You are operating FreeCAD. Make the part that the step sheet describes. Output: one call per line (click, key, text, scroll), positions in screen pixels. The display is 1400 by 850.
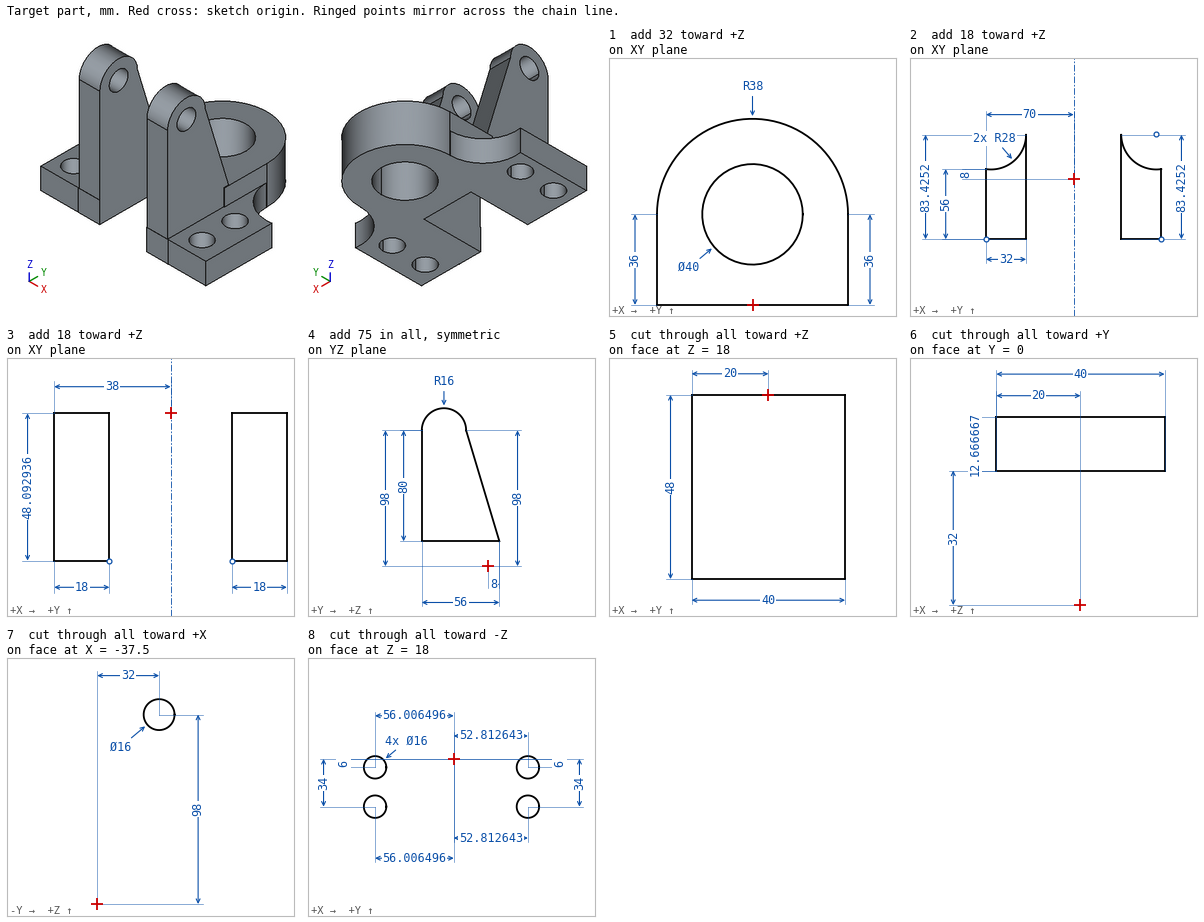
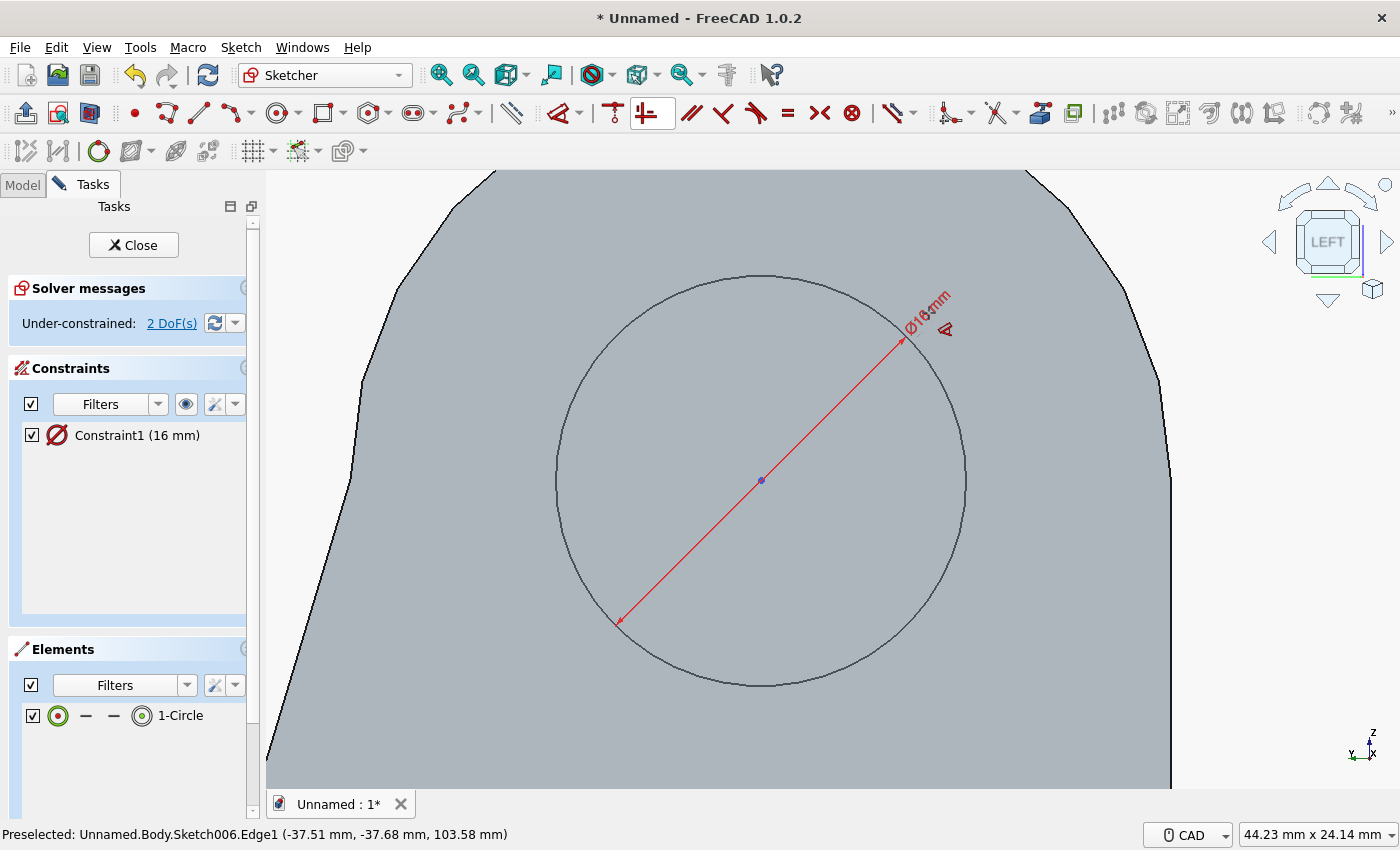
click(761, 481)
click(527, 447)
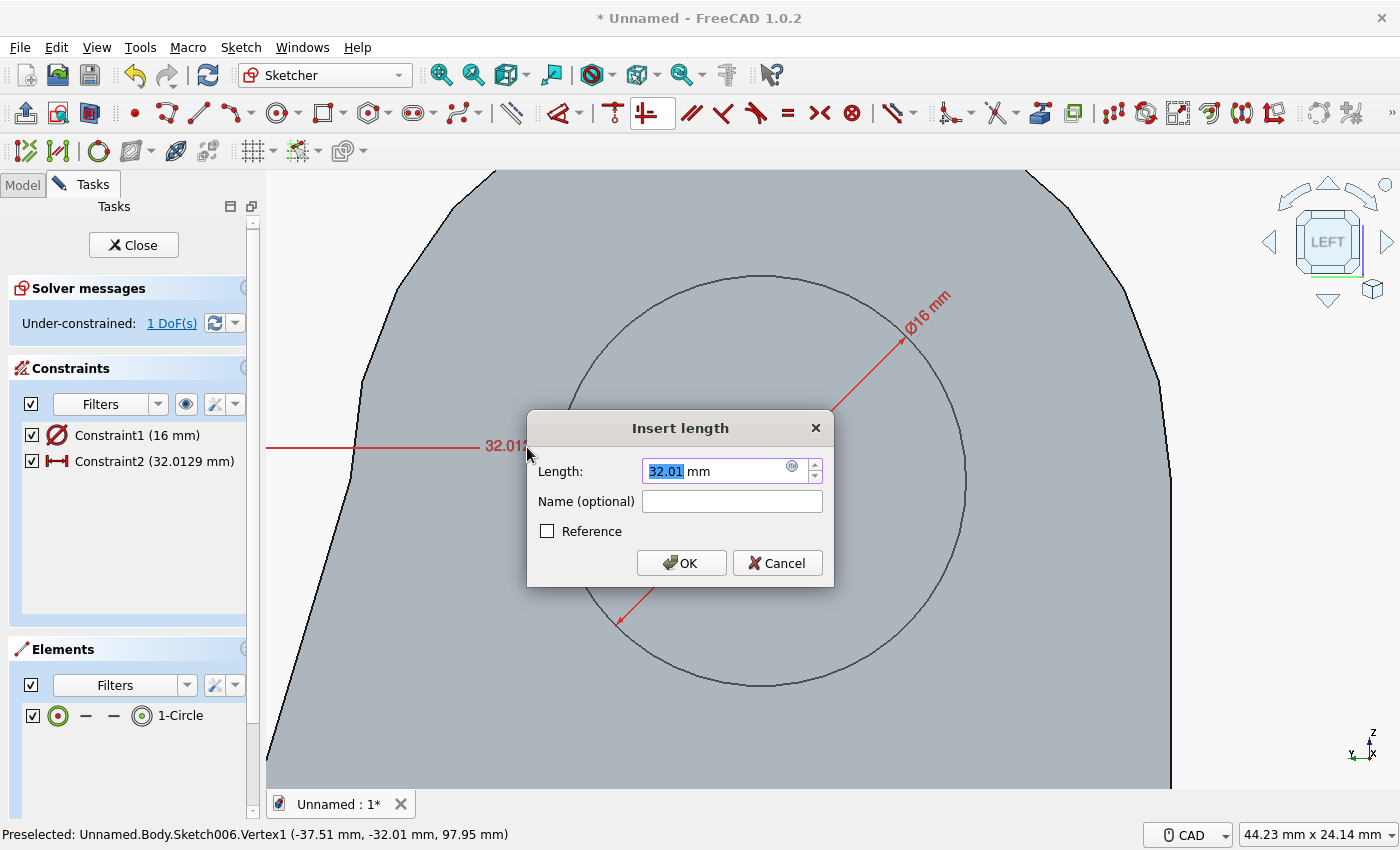
text(32)
key(Return)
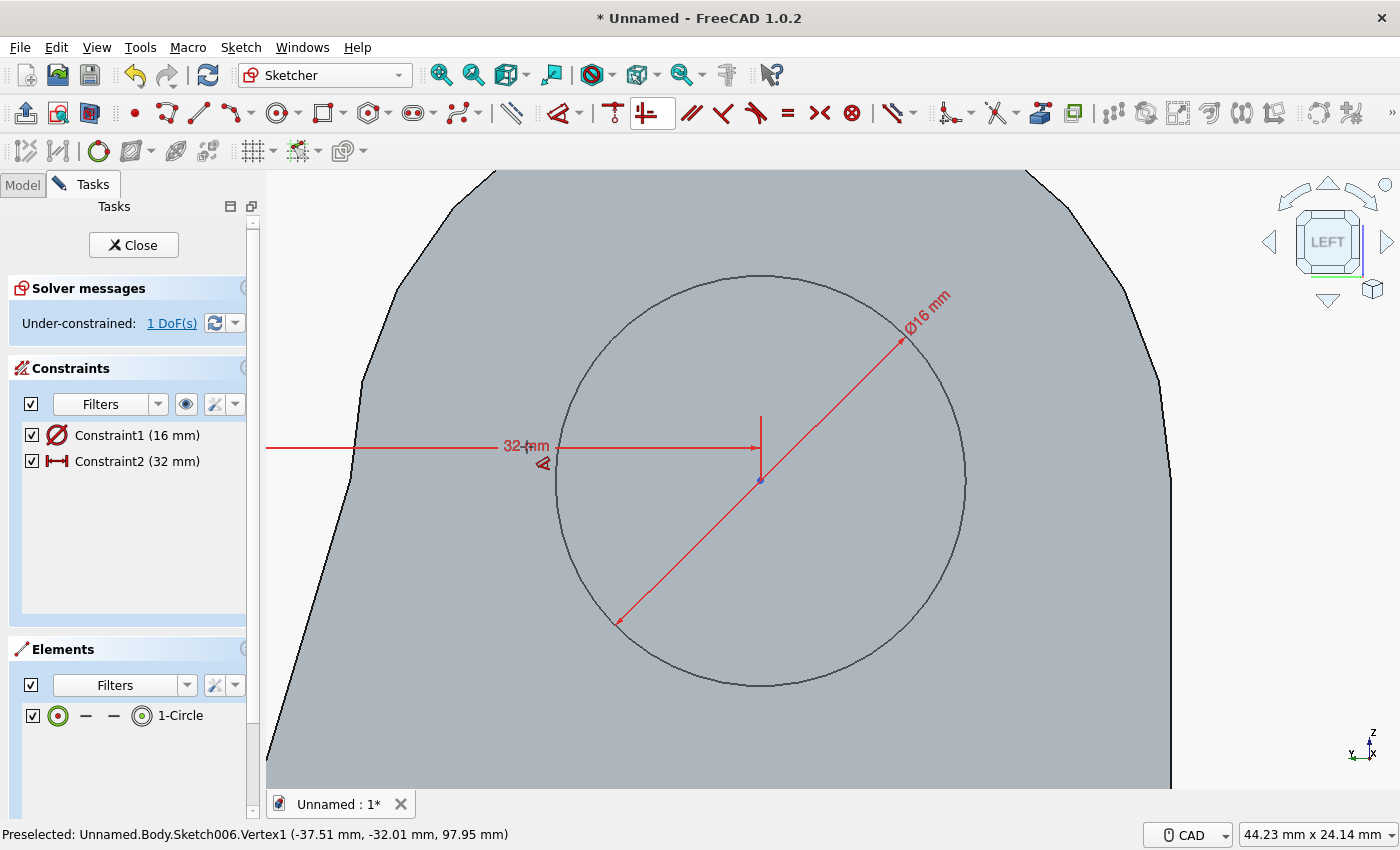
click(761, 481)
click(795, 621)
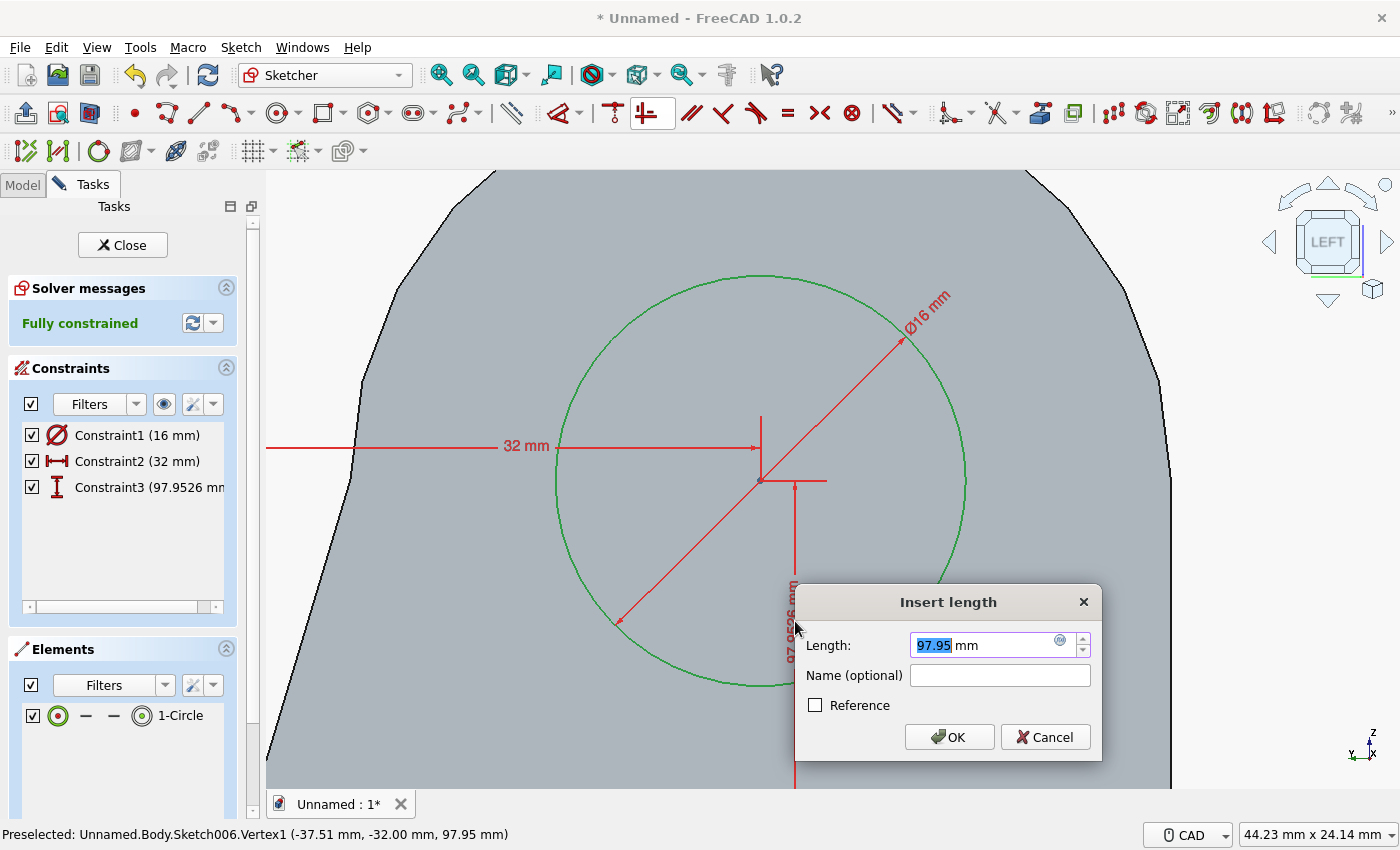
text(98)
key(Return)
key(Escape)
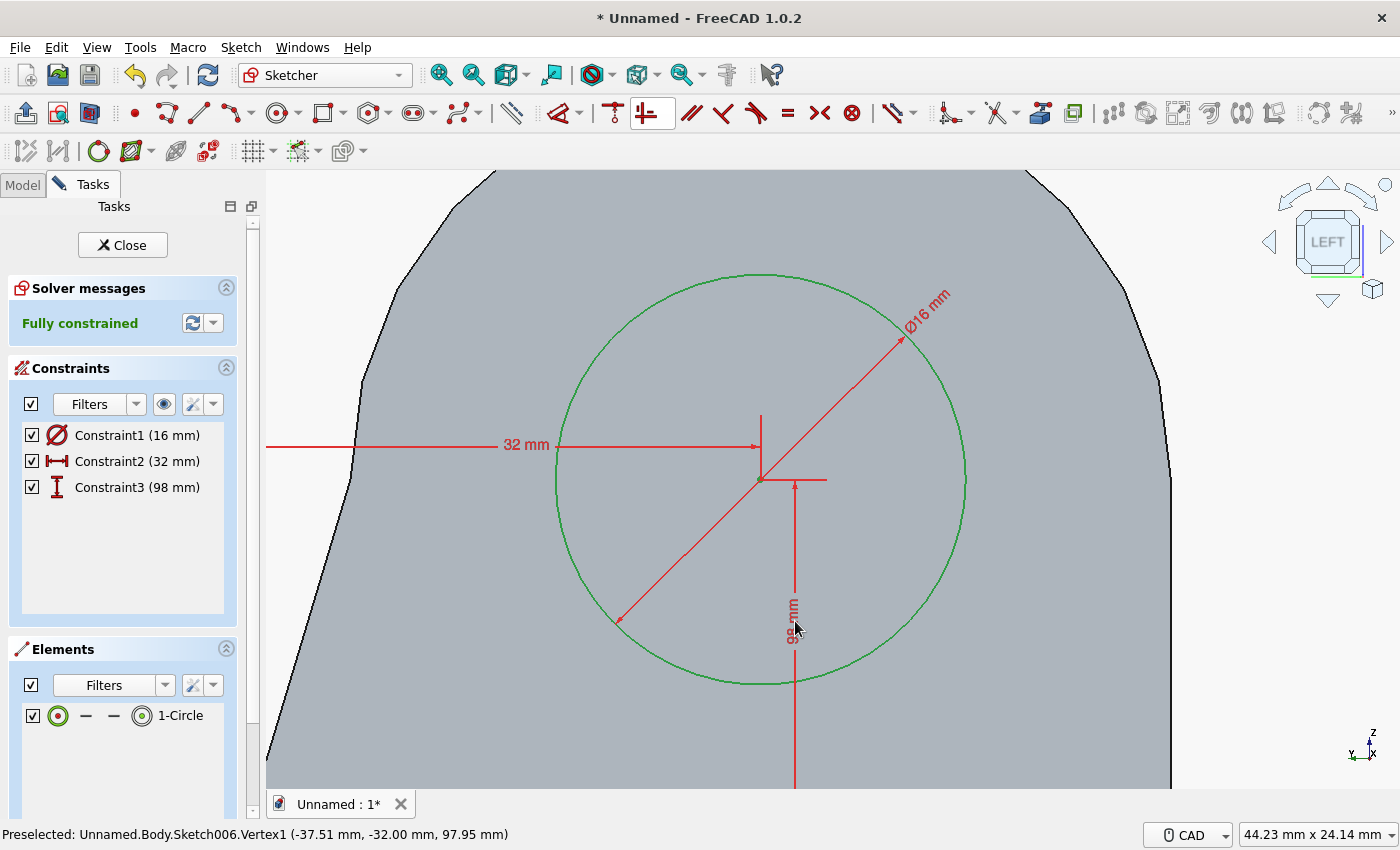
click(123, 245)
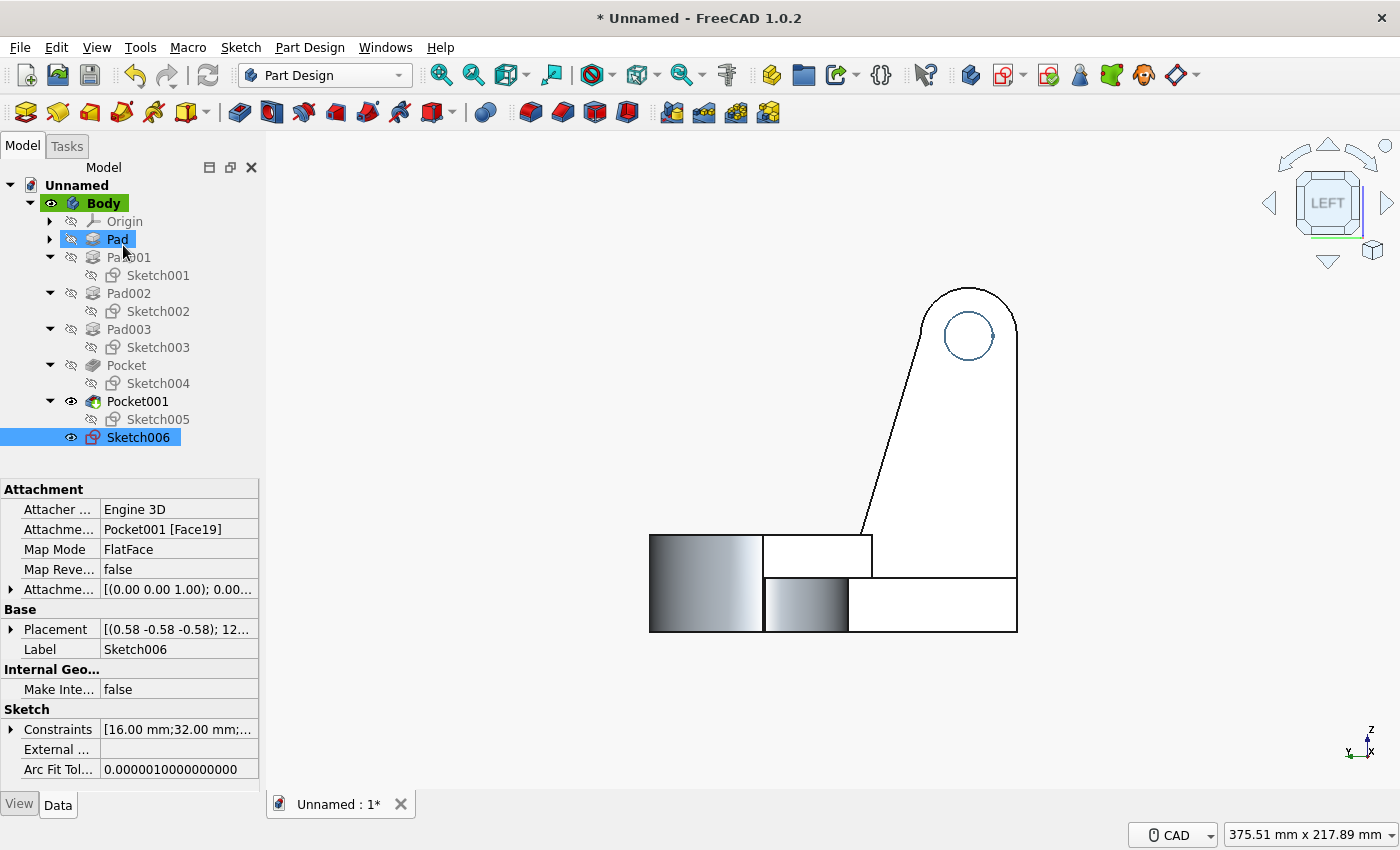
click(240, 112)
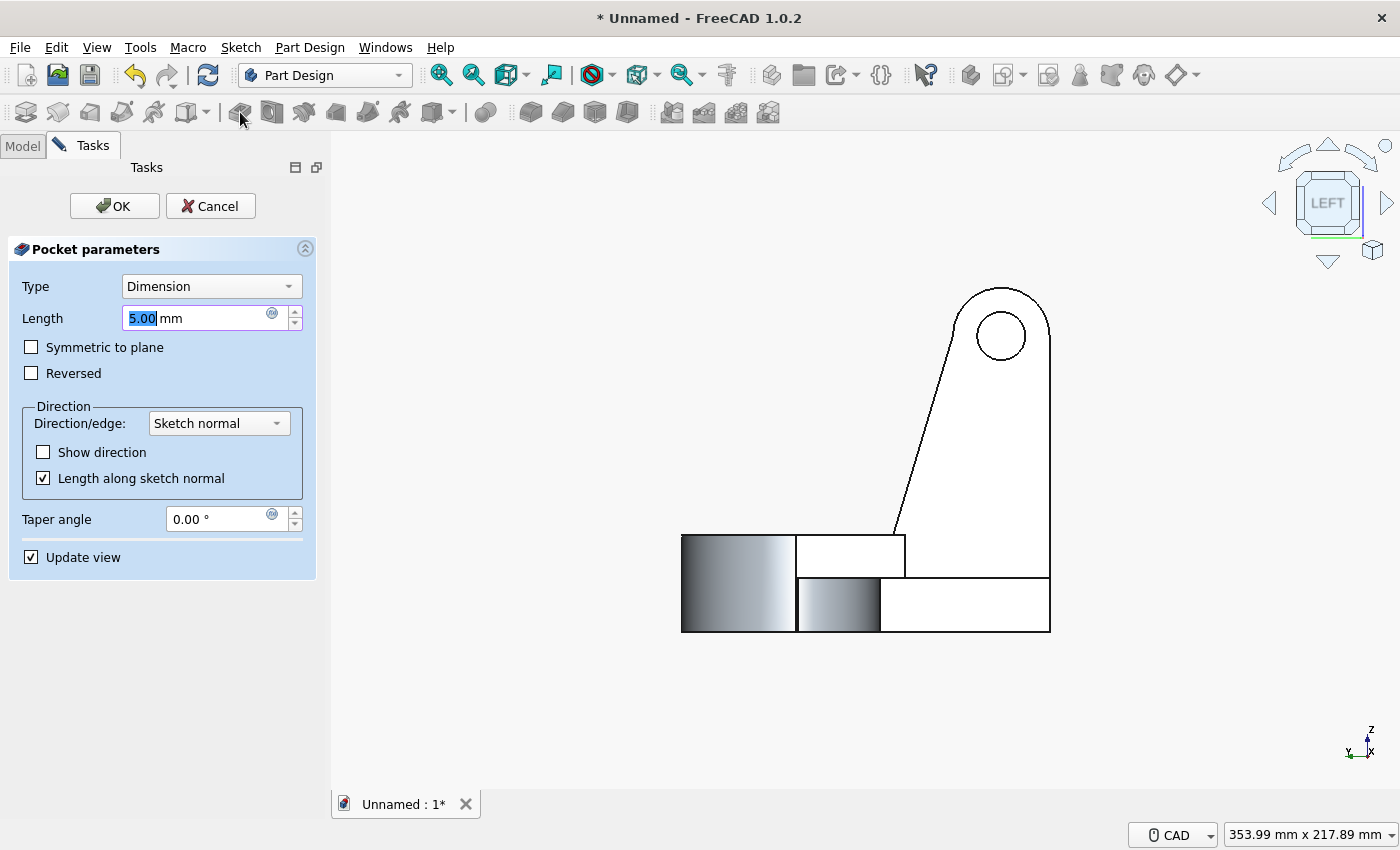
click(212, 286)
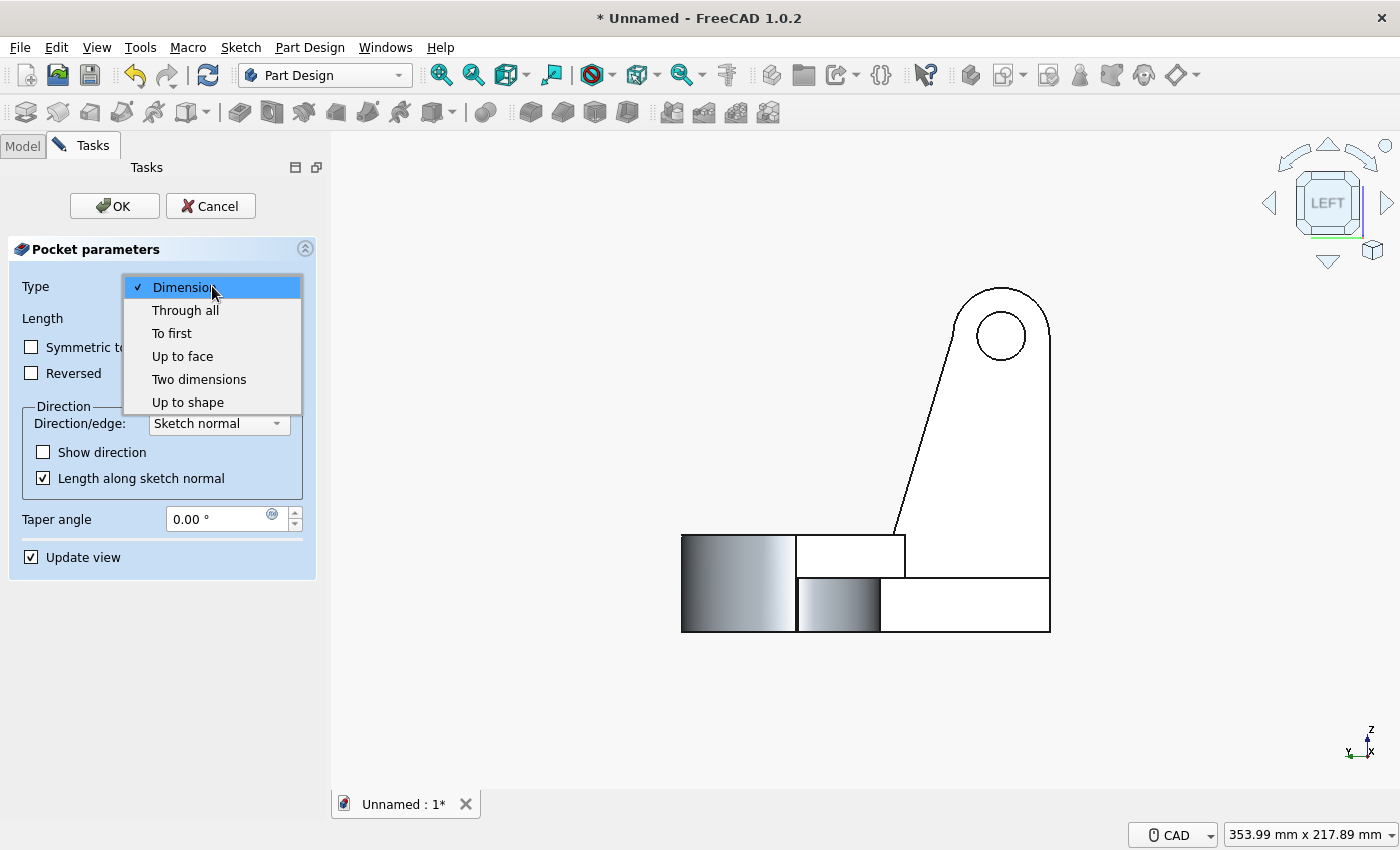
click(212, 310)